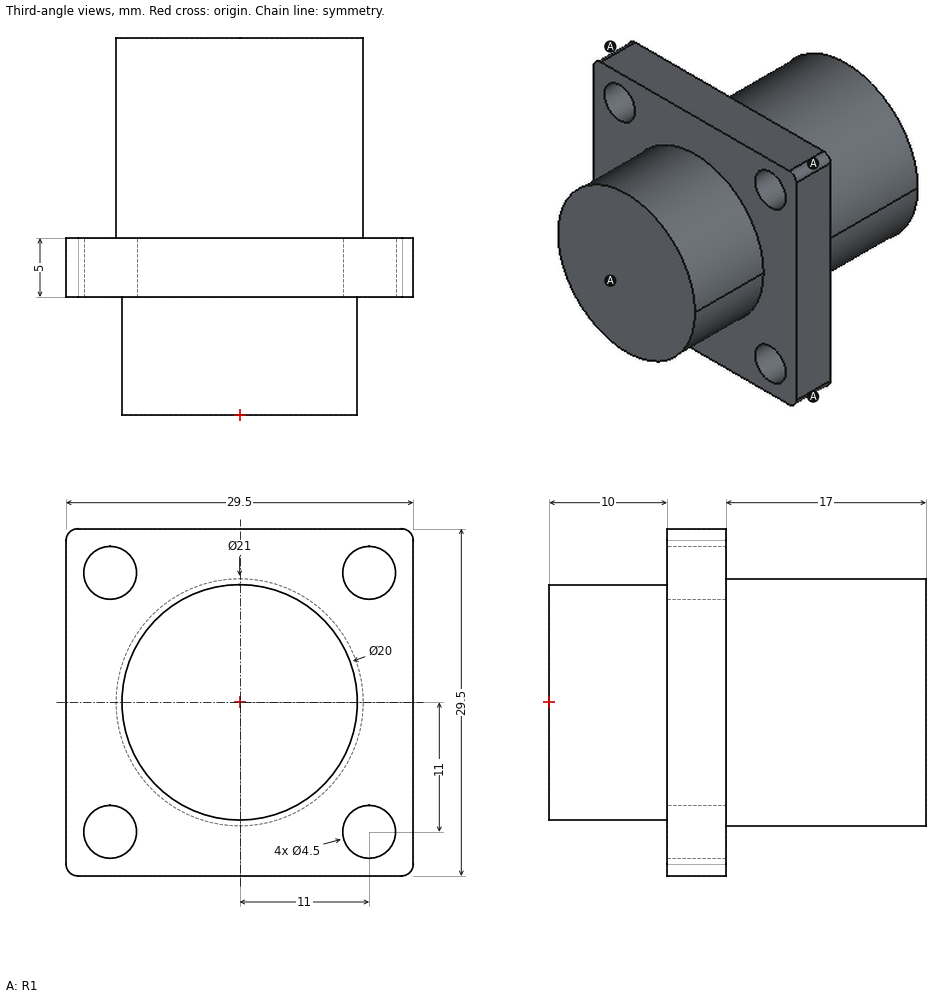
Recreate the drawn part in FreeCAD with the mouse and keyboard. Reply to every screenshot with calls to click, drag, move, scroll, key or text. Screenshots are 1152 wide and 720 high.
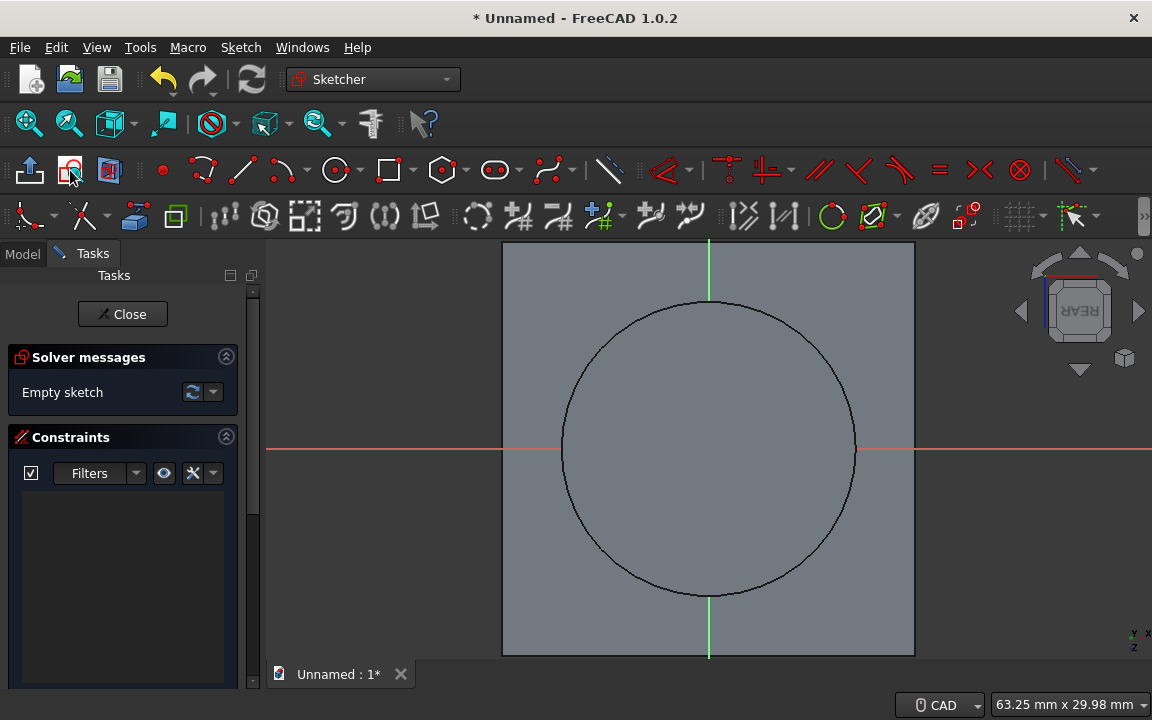
scroll(502, 449, down, 2)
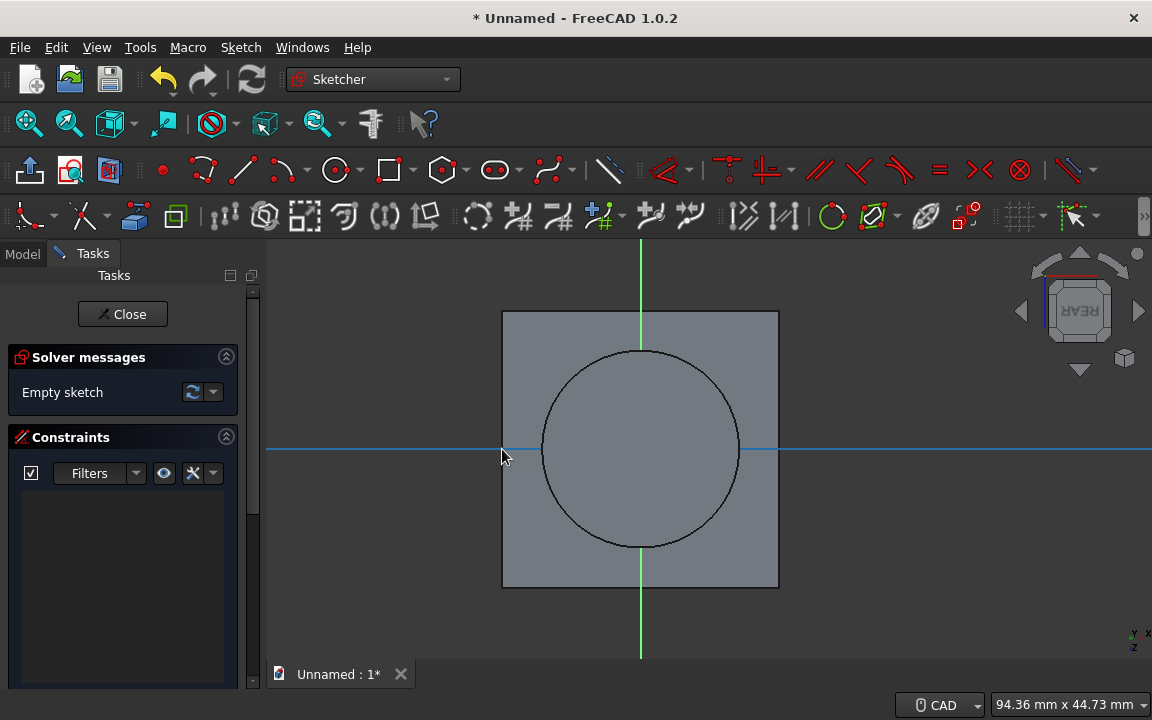
click(336, 170)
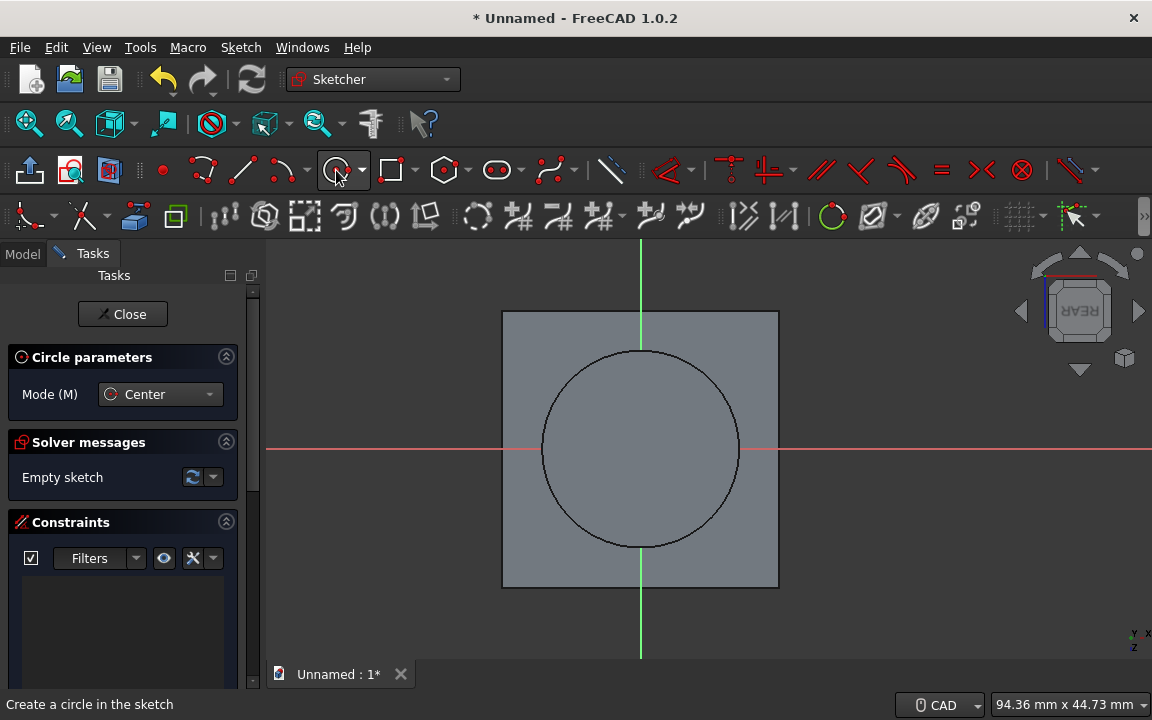
click(744, 346)
move(759, 331)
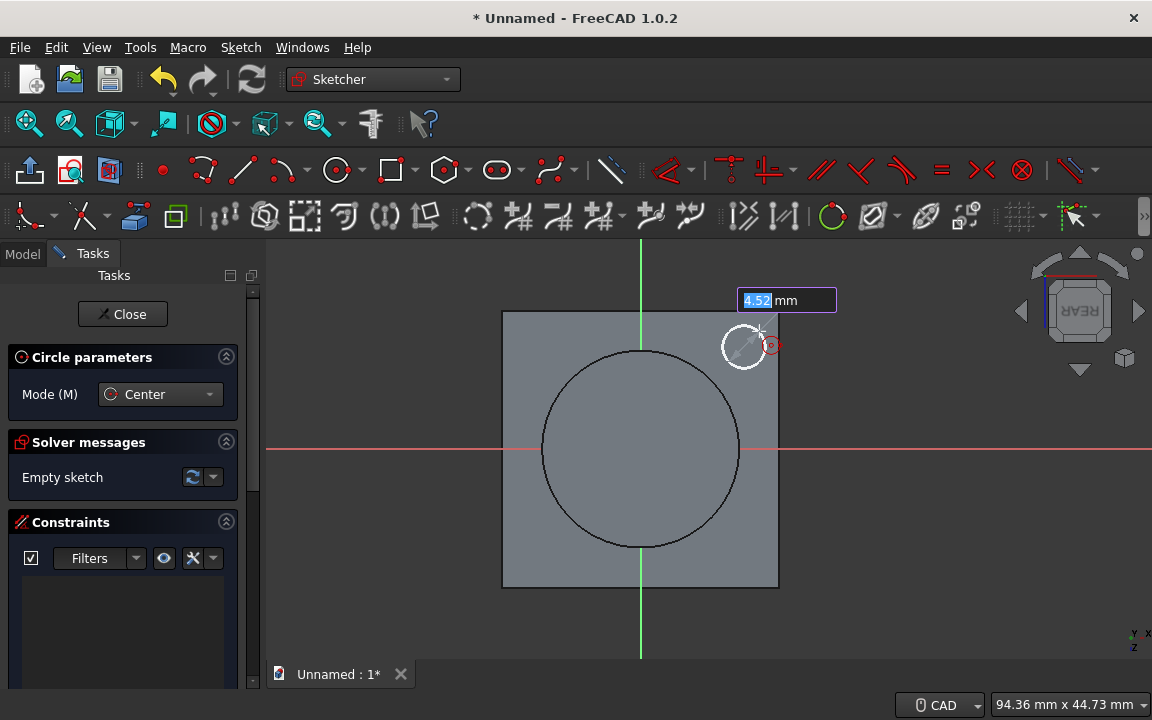
text(4.5)
key(Return)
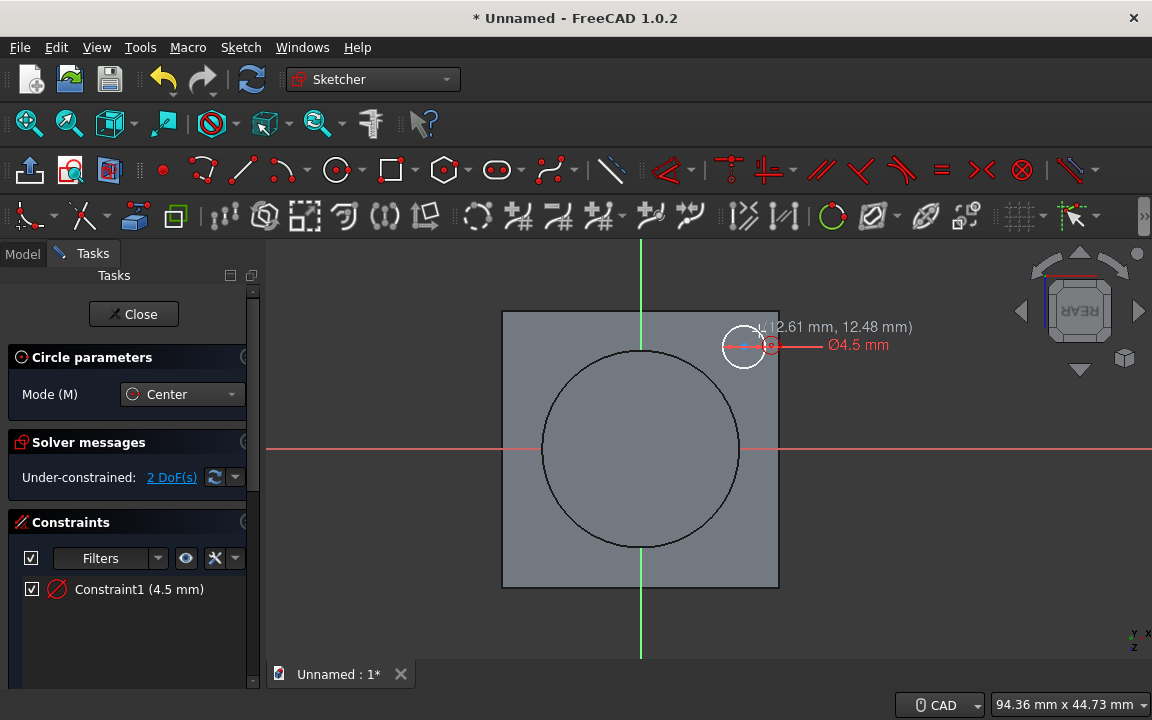
click(537, 346)
move(552, 331)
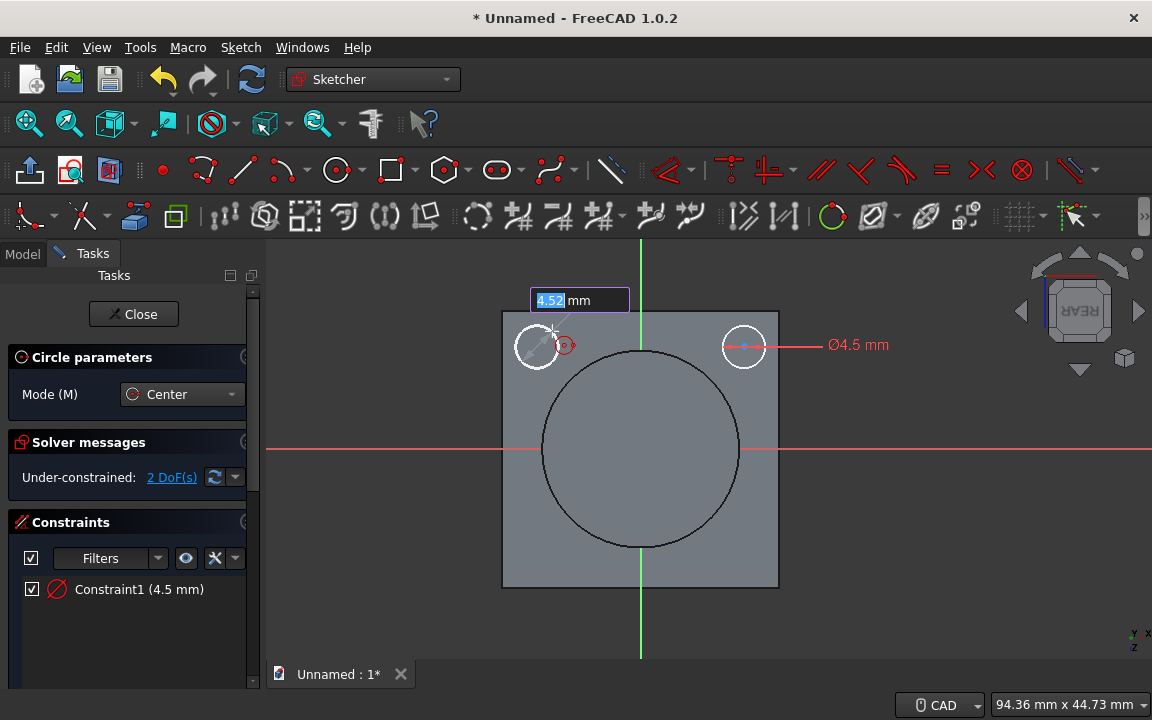
text(4.5)
key(Return)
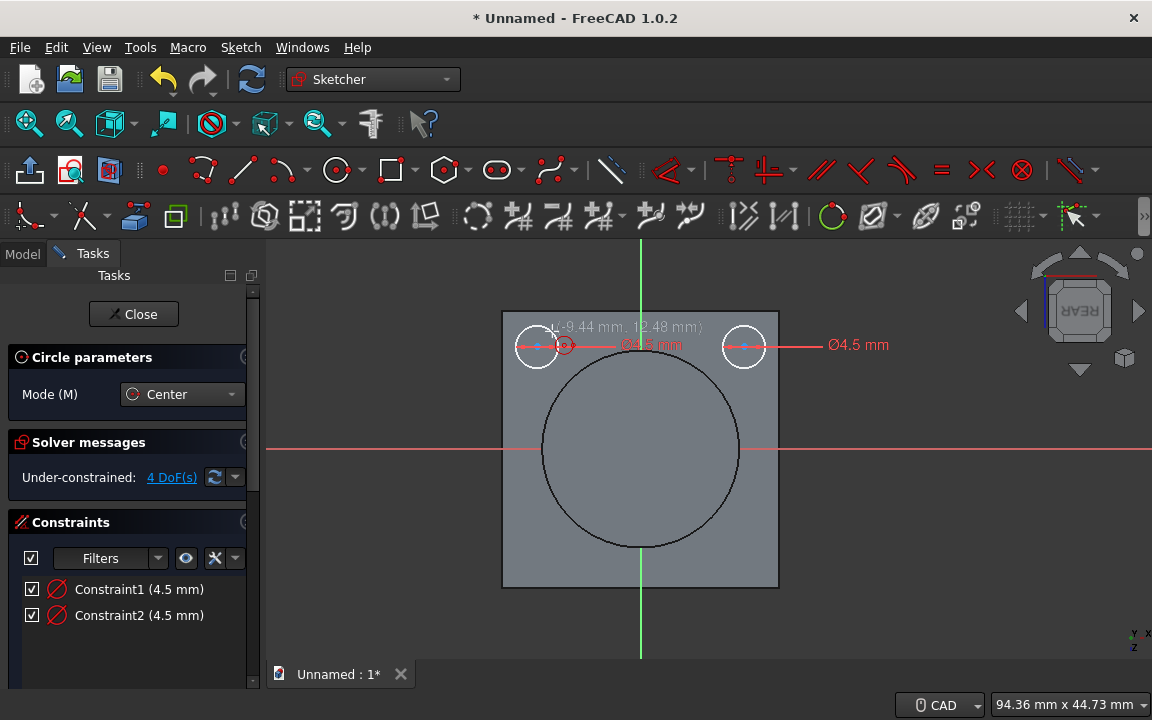
click(537, 552)
move(552, 538)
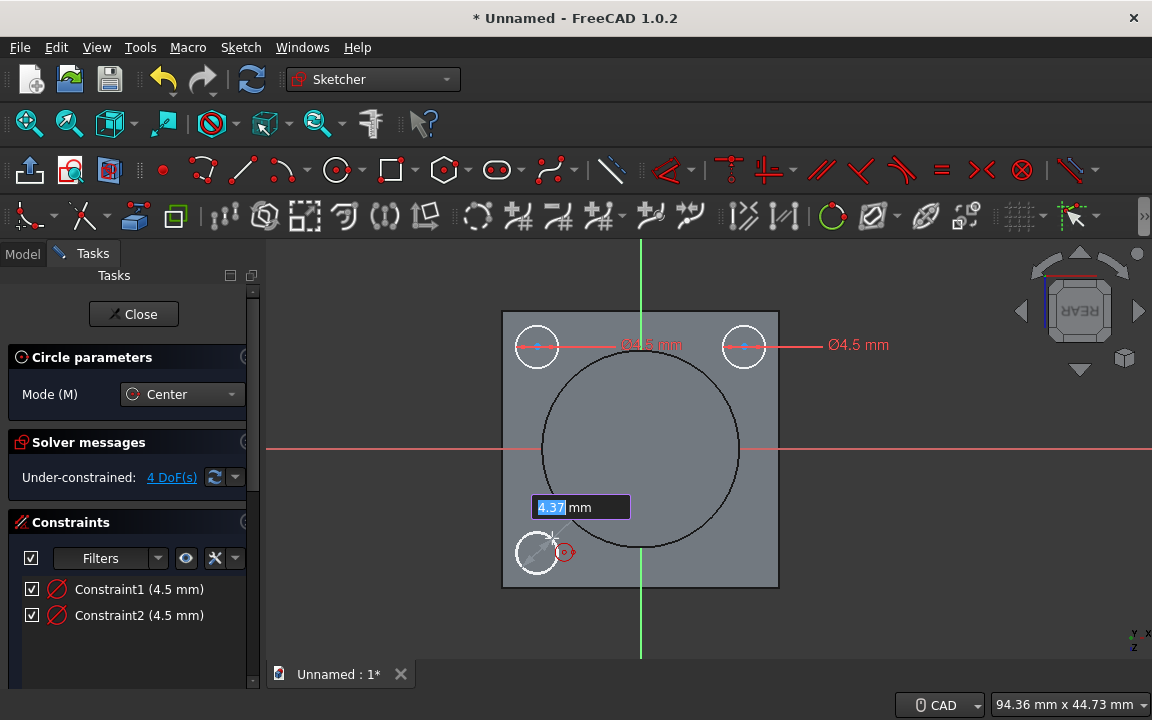
text(4.5)
key(Return)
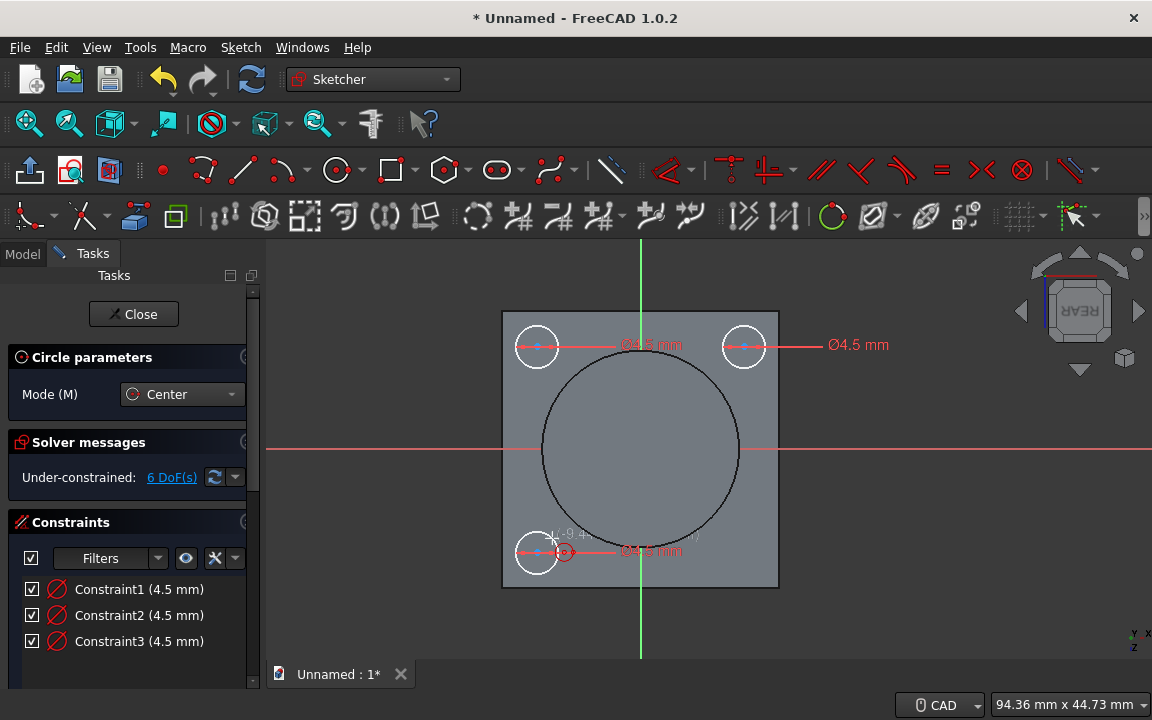
click(744, 552)
move(759, 538)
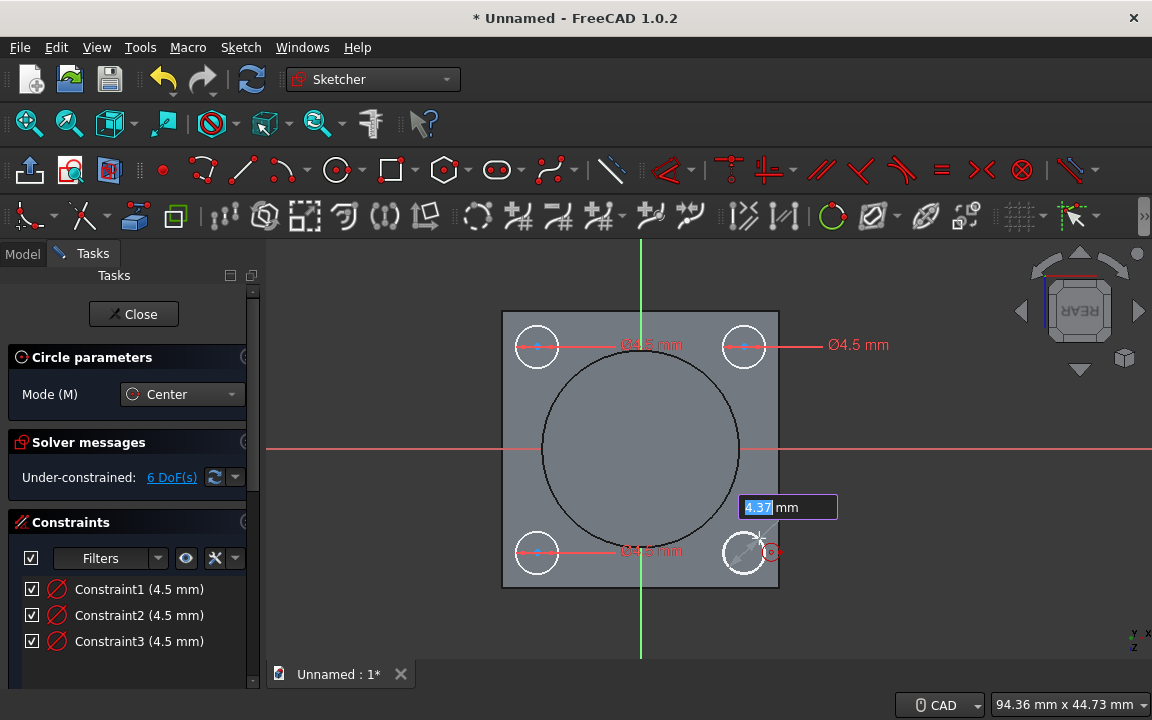
text(4.5)
key(Return)
key(Escape)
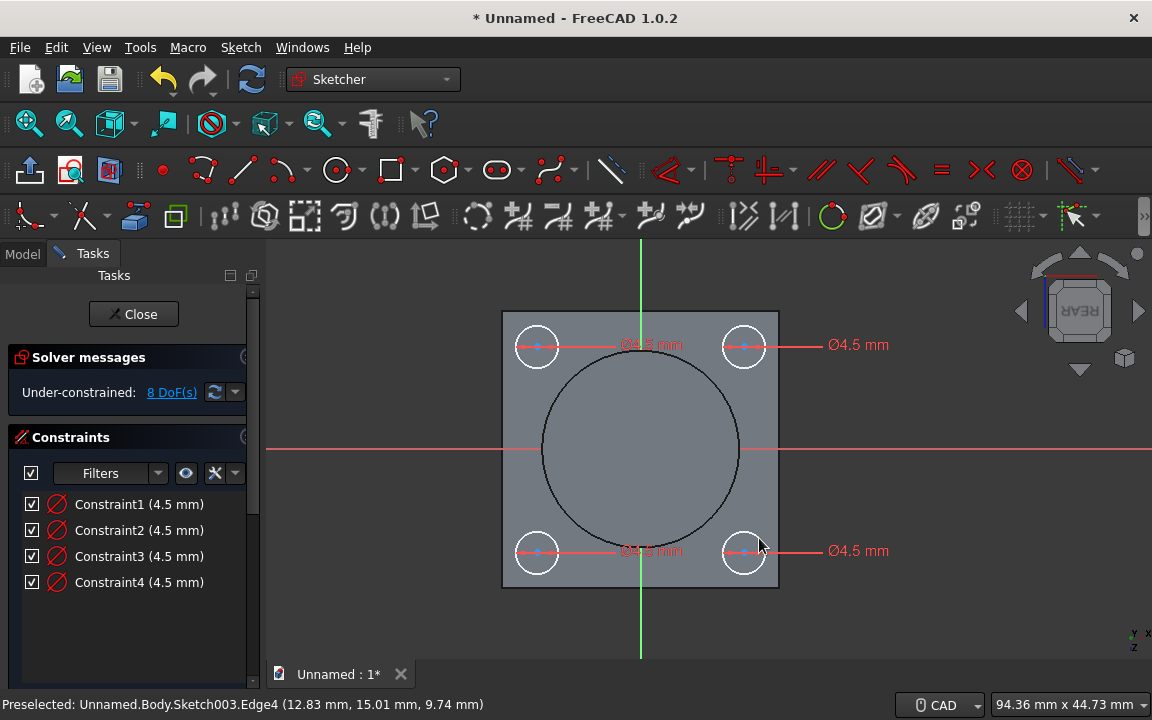
click(744, 347)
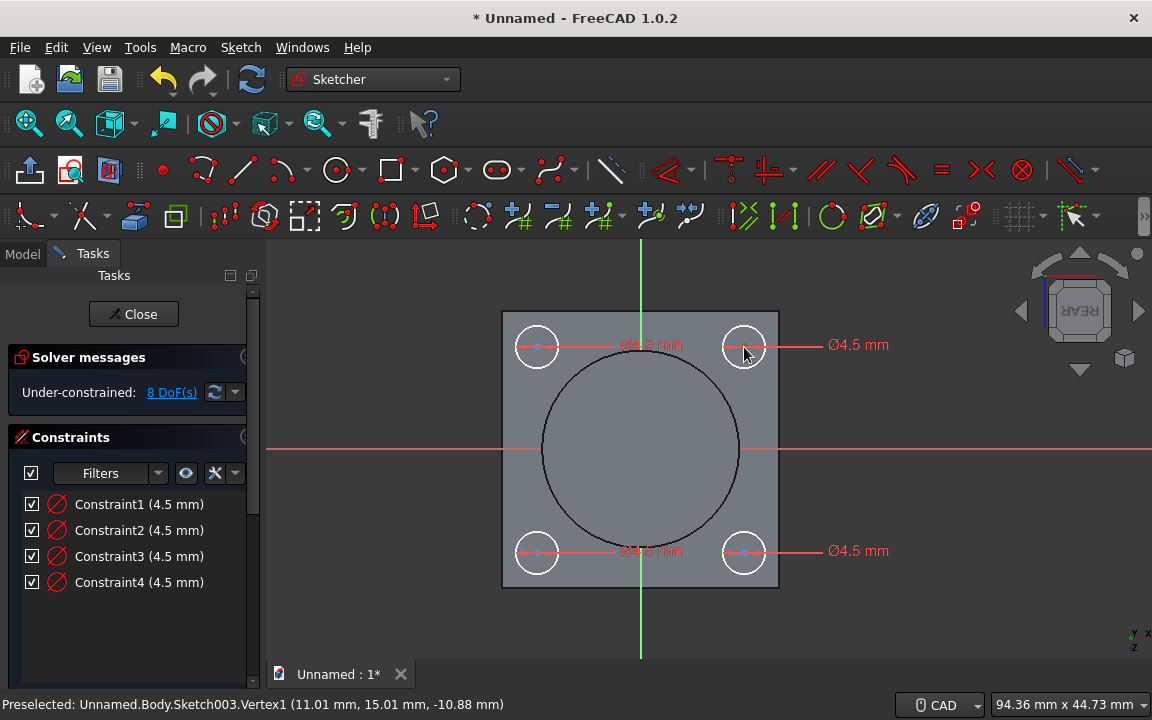
click(537, 347)